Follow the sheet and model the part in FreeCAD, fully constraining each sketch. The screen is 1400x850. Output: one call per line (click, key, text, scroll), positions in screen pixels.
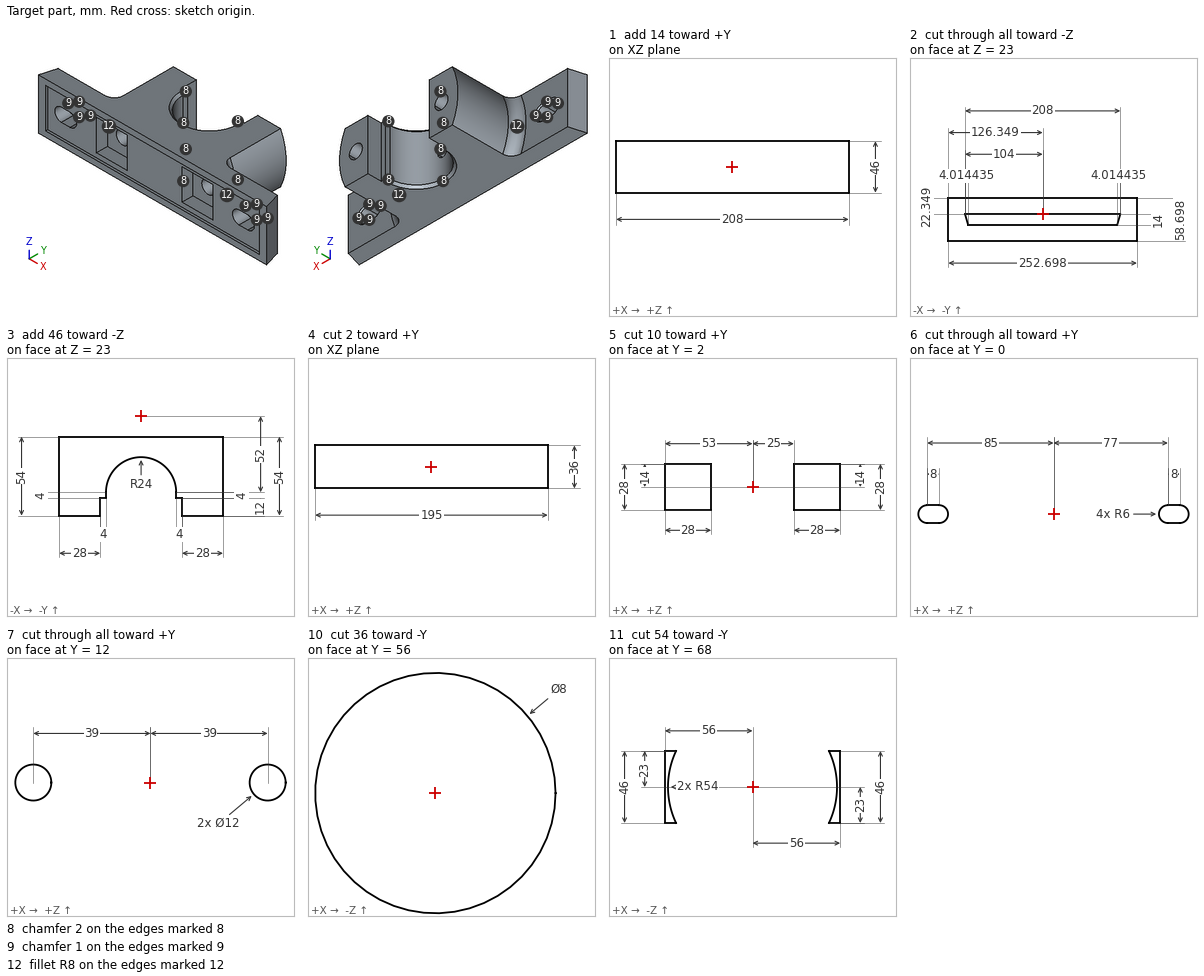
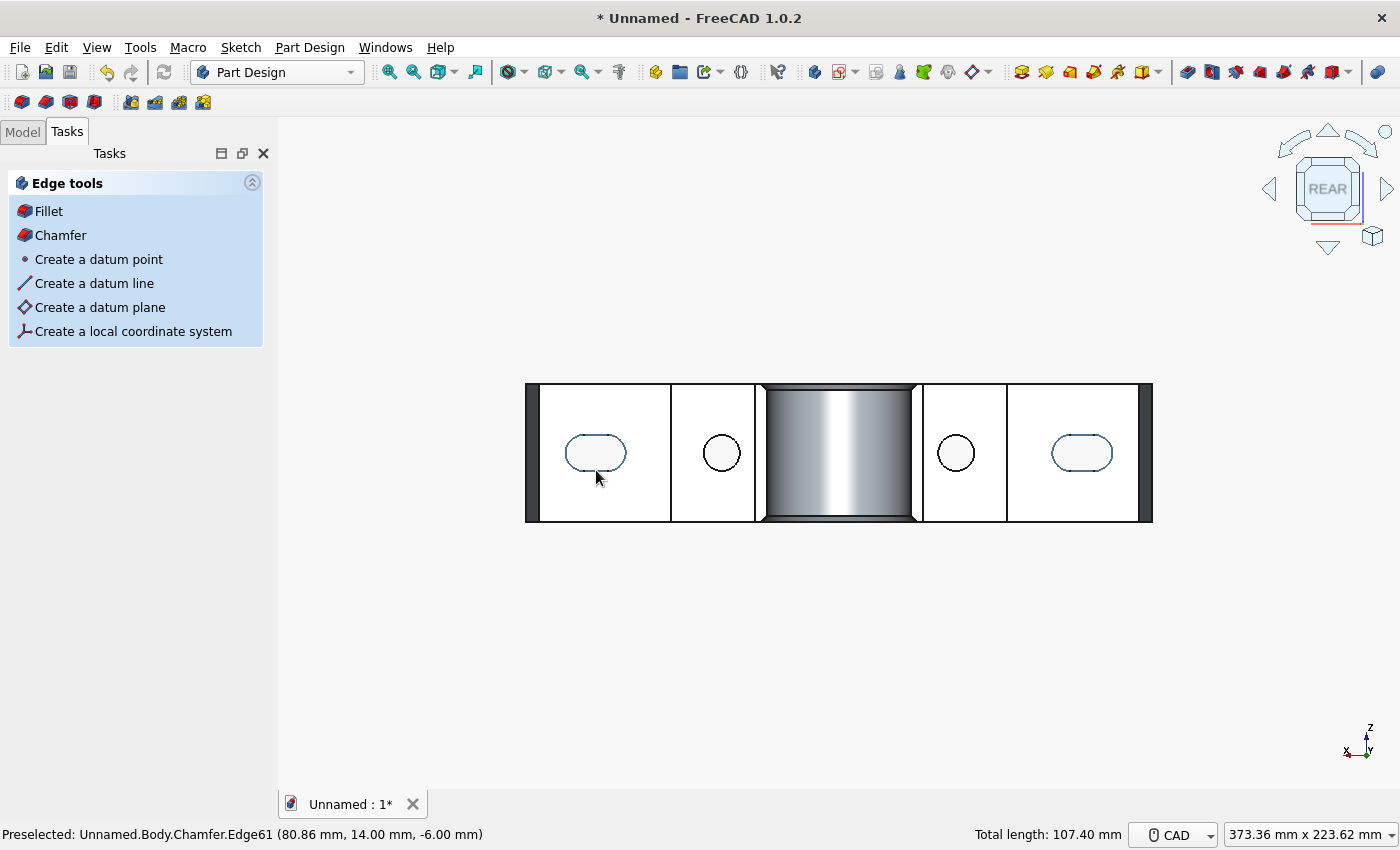
click(46, 102)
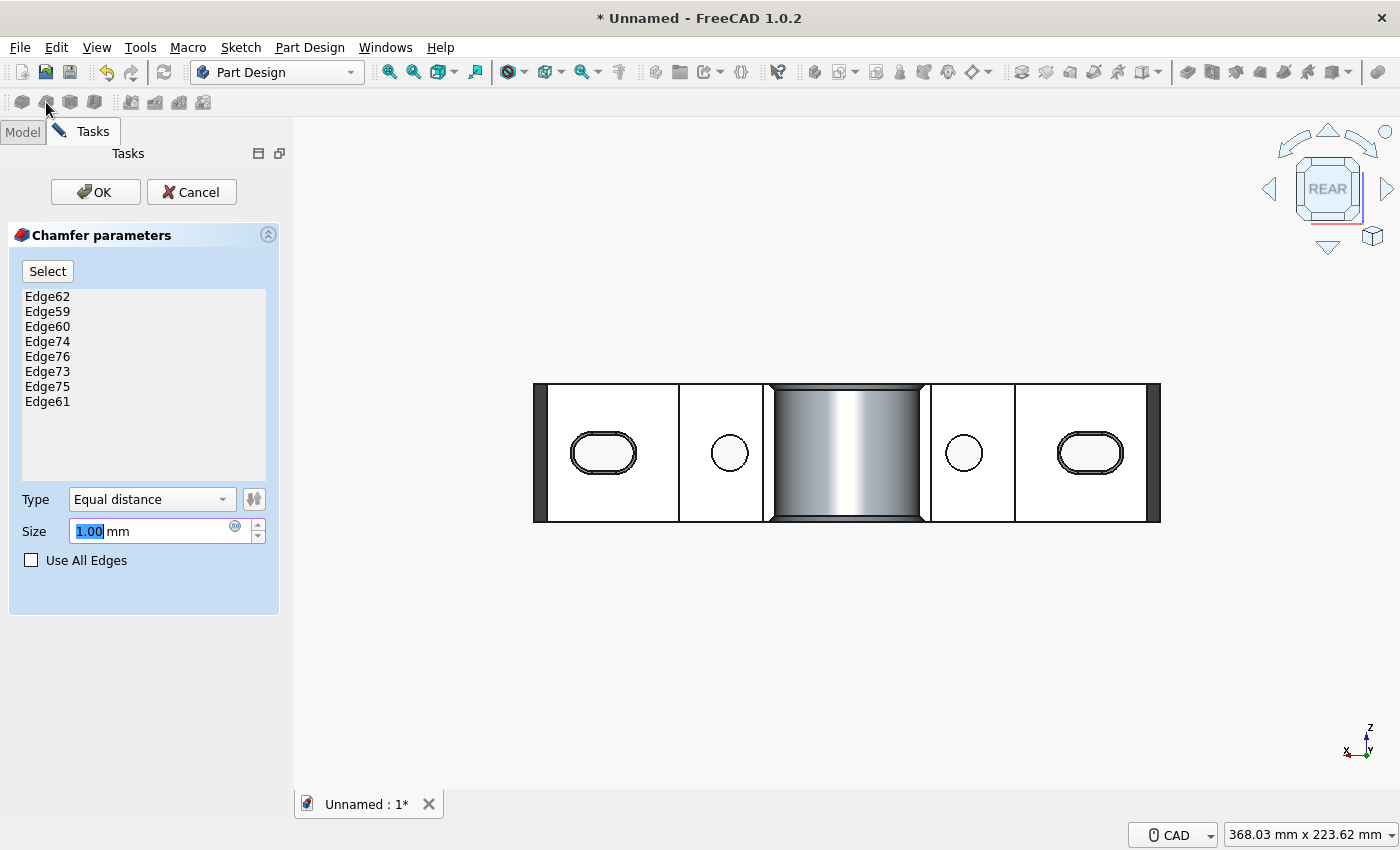
text(1)
key(Tab)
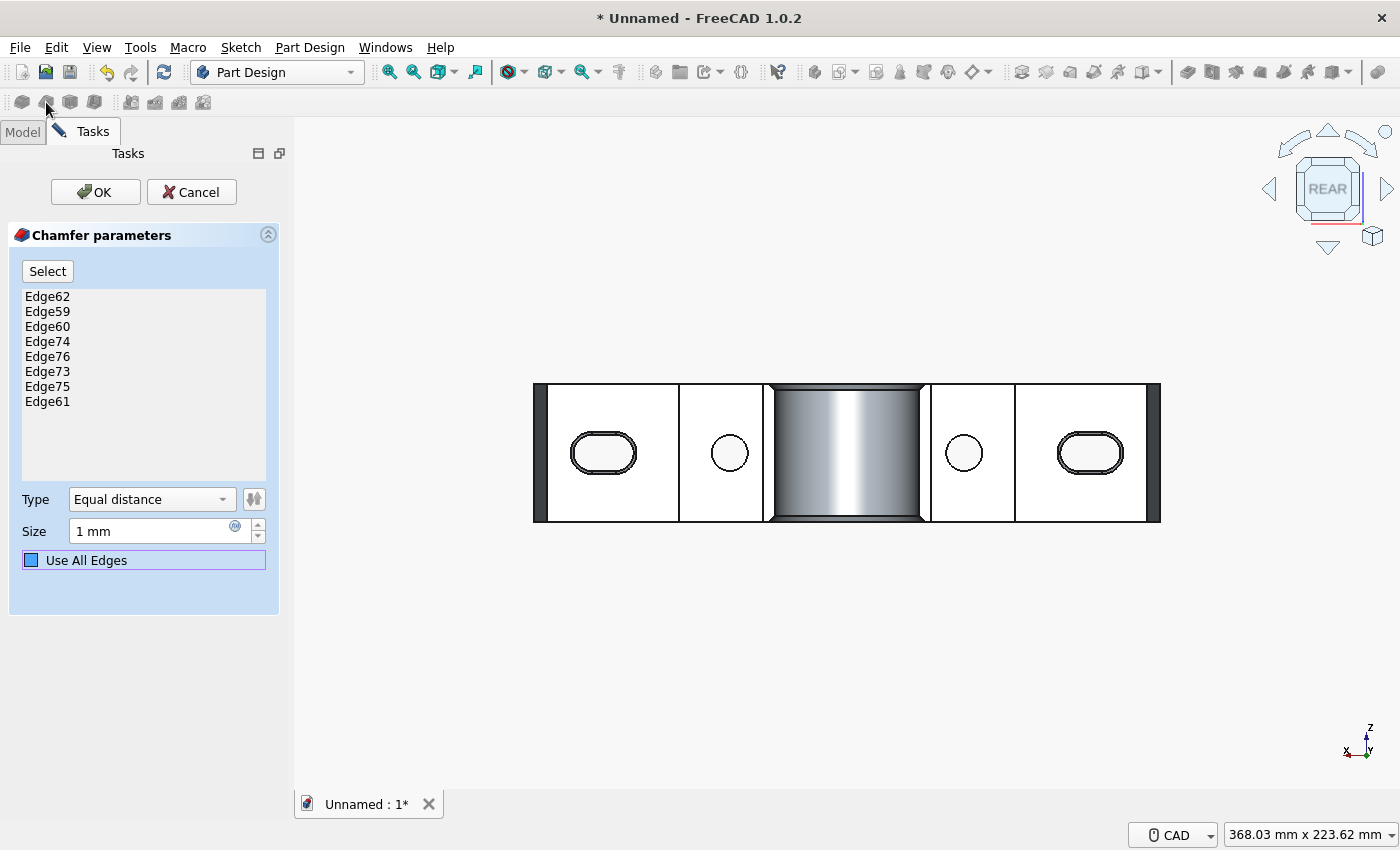
click(96, 192)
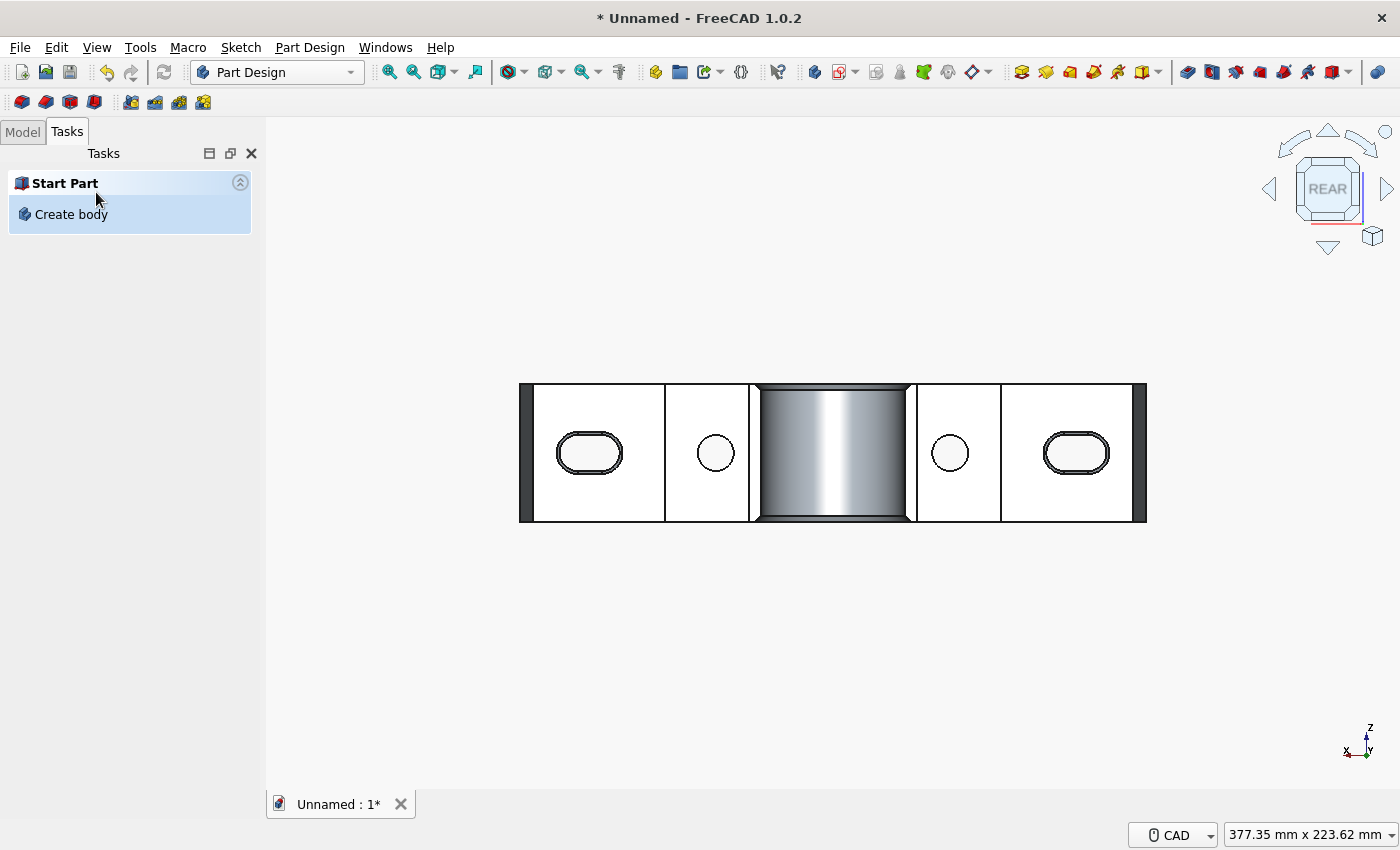
scroll(755, 413, up, 4)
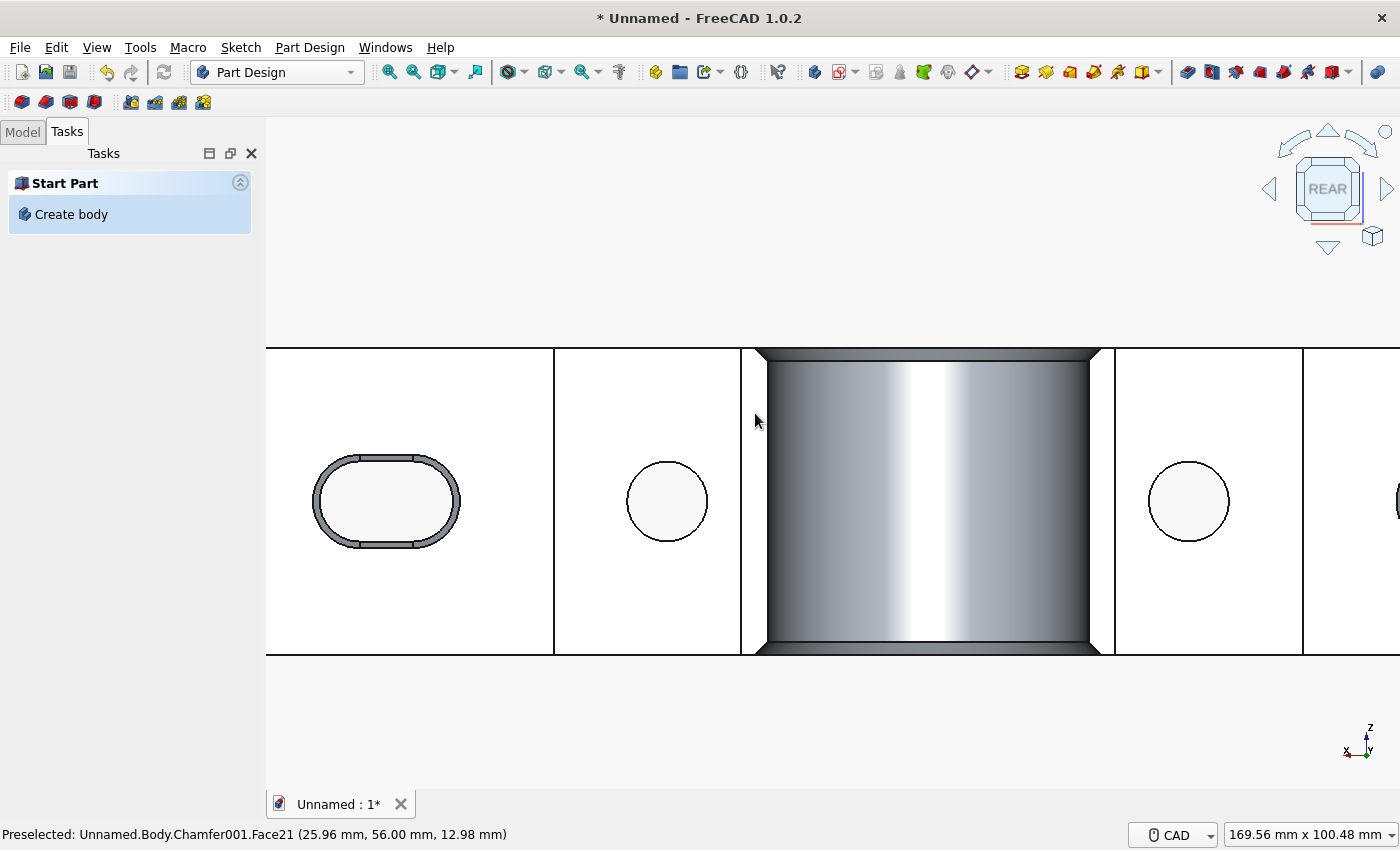
click(754, 413)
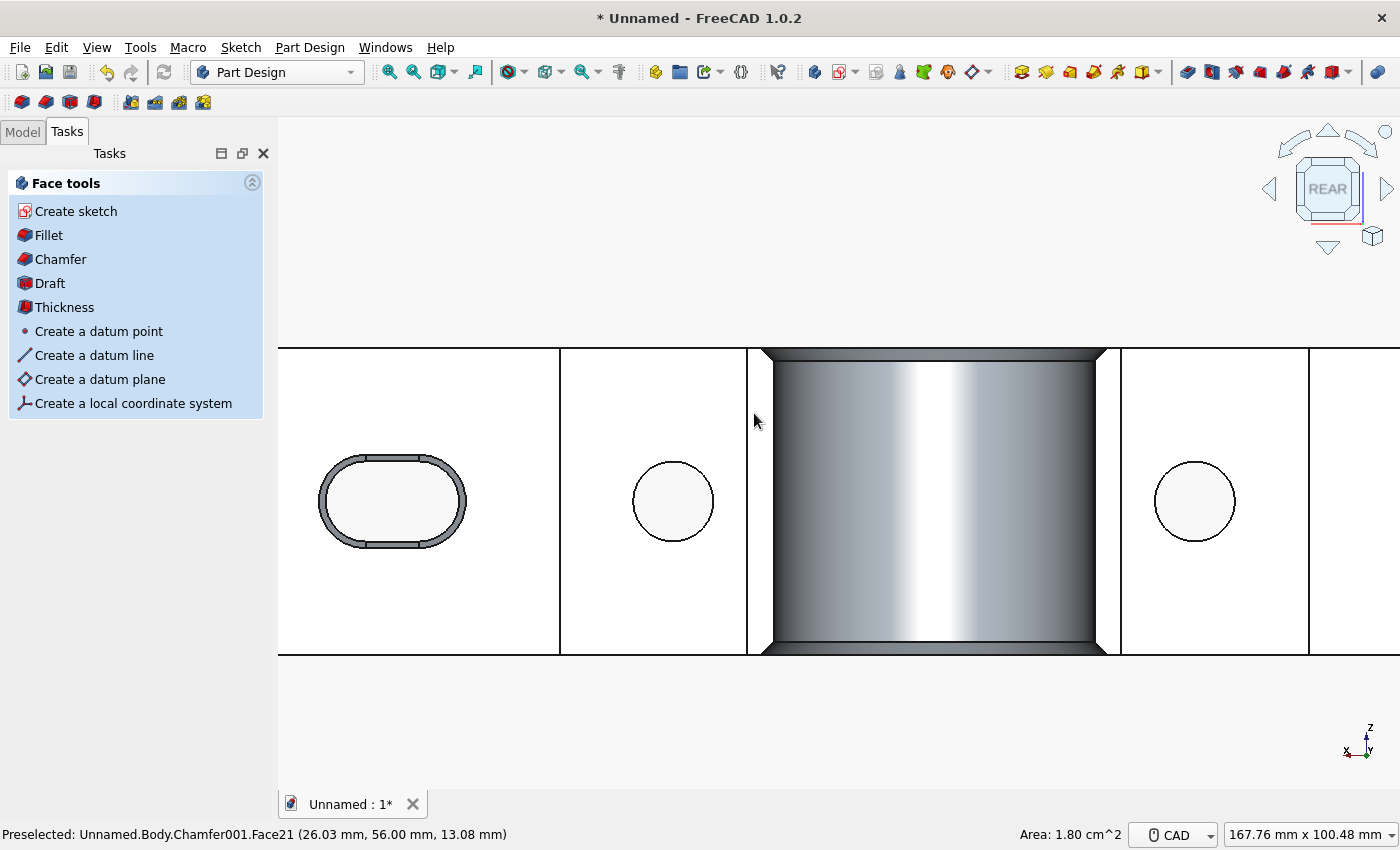
click(840, 72)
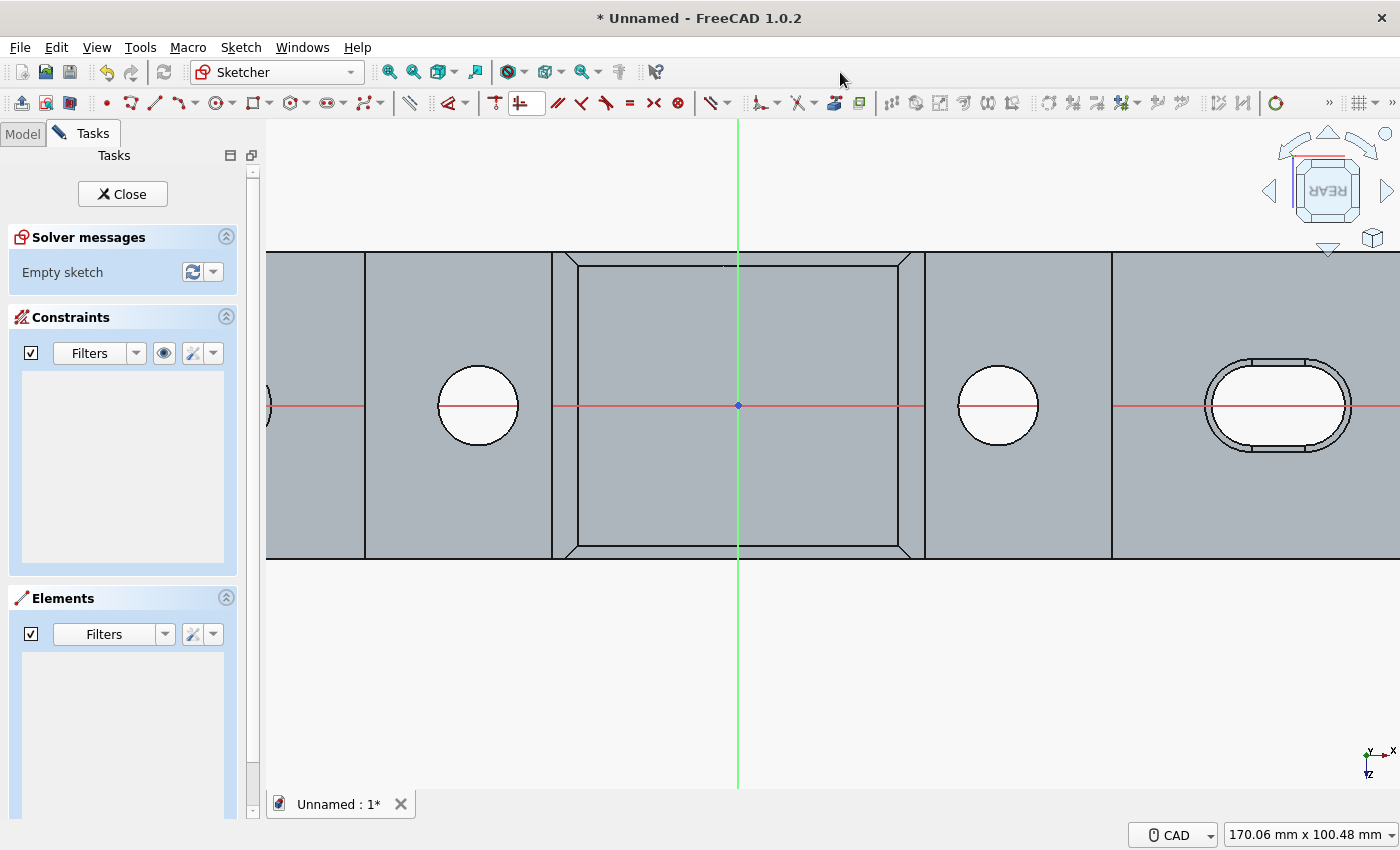
key(q)
key(s)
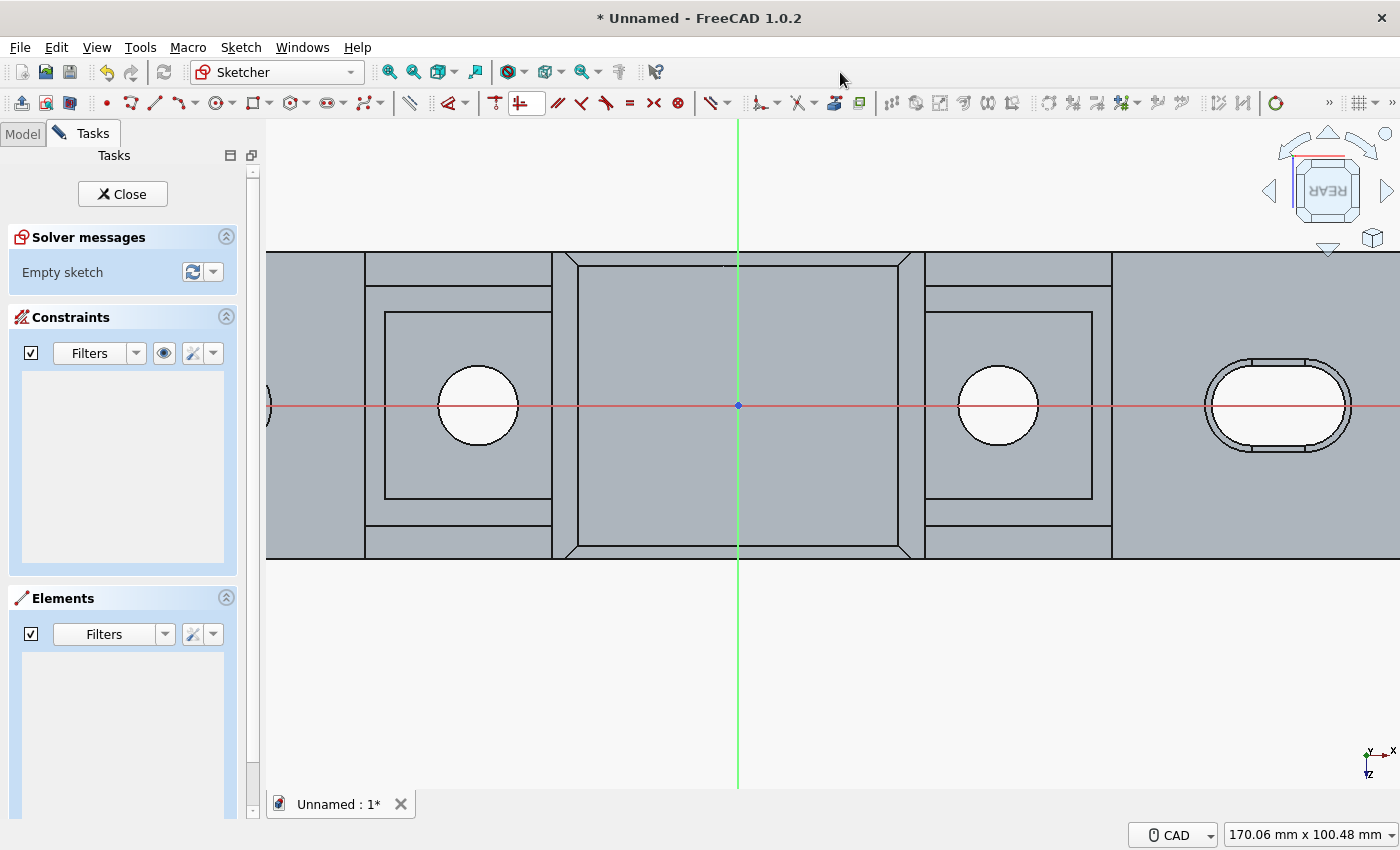
scroll(734, 398, up, 10)